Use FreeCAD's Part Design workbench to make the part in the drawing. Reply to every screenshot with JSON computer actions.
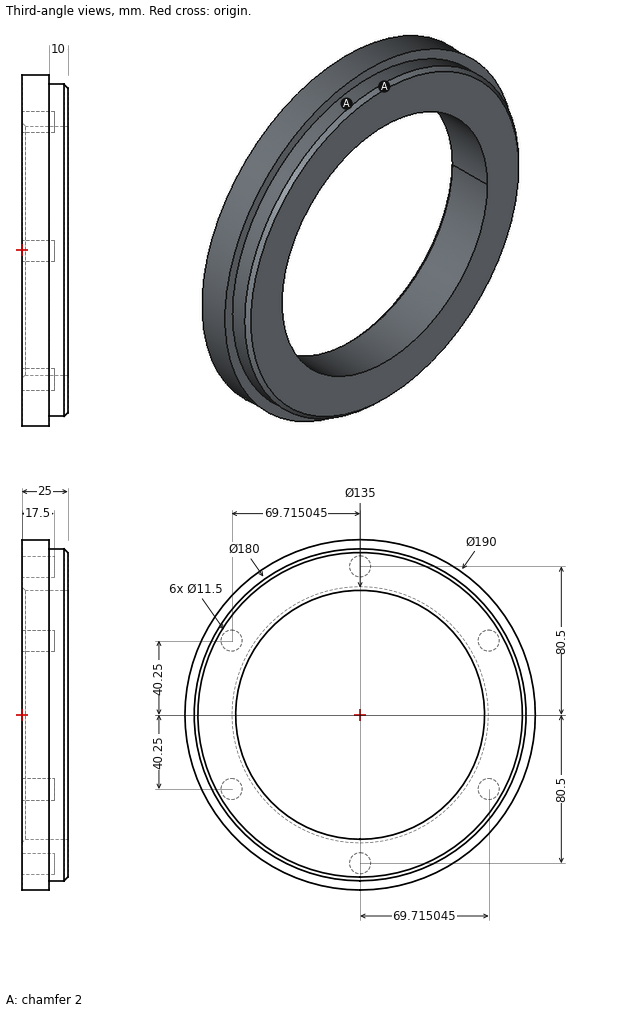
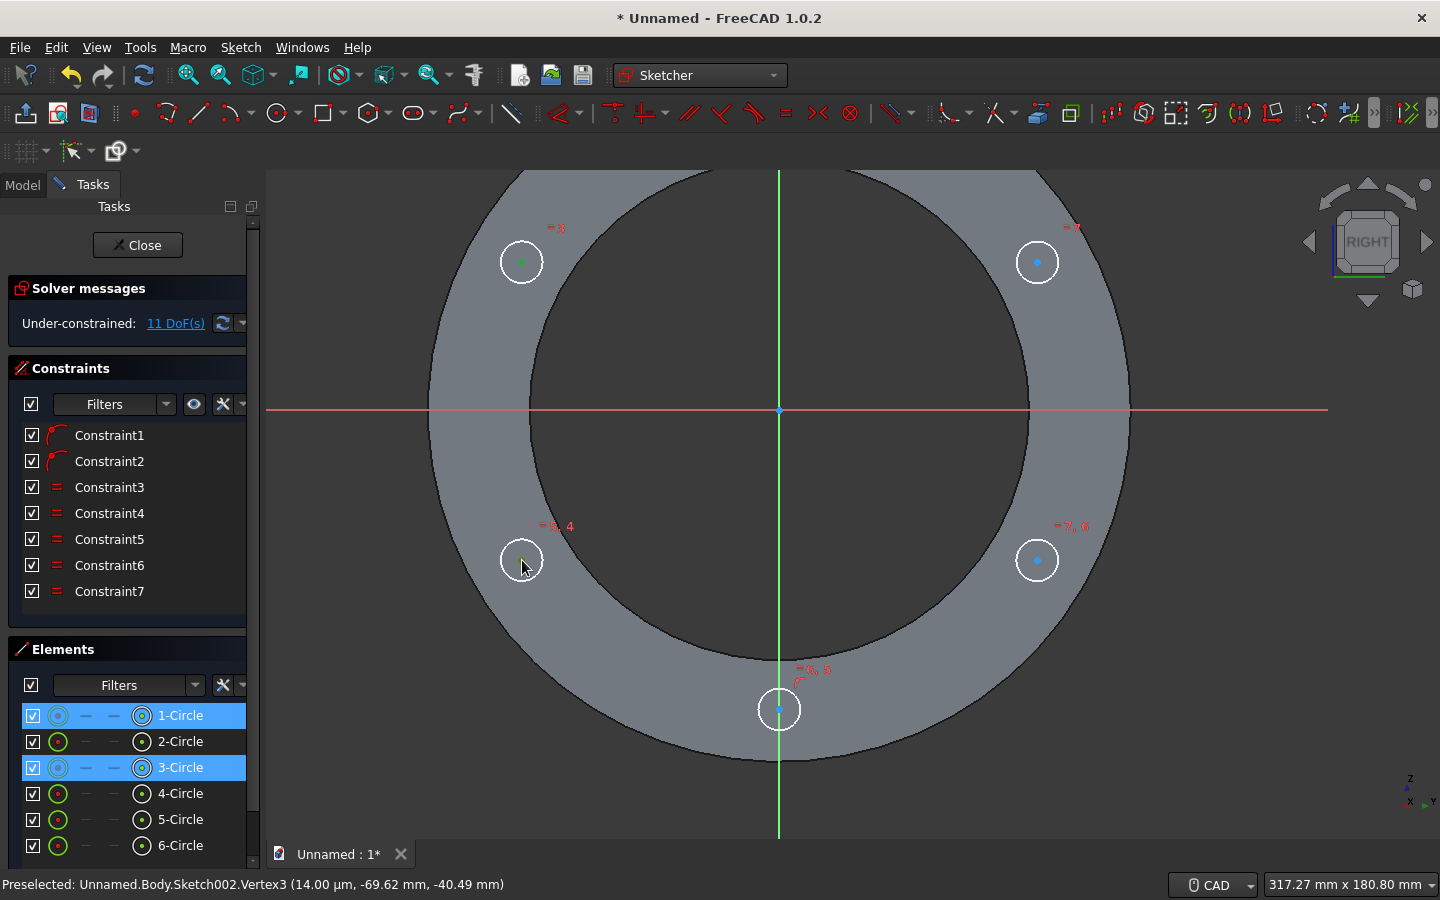
{"action": "key", "text": "v"}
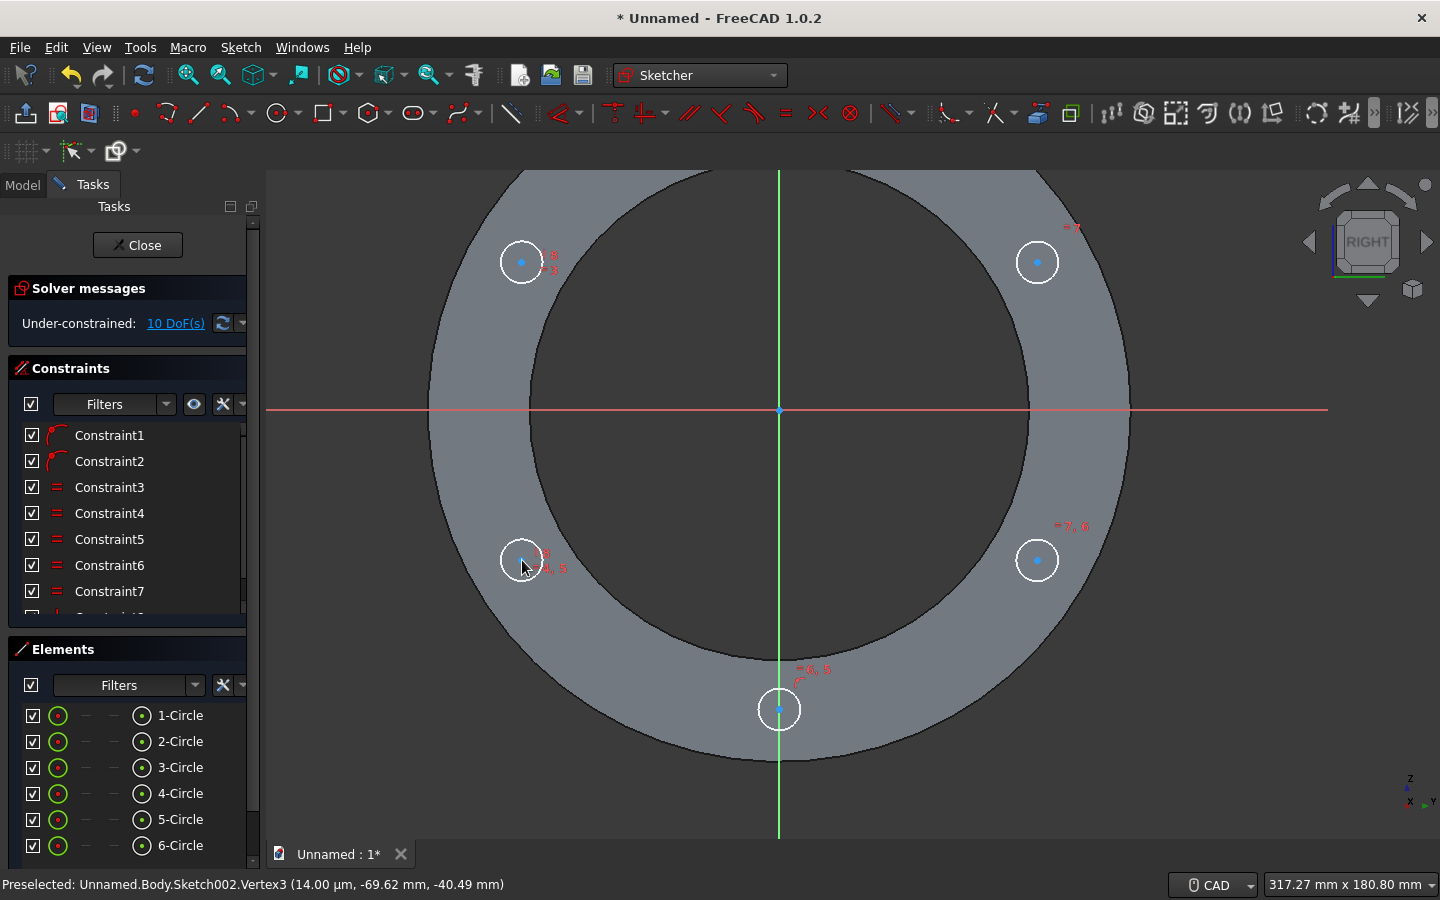
{"action": "left_click", "coordinate": [522, 560]}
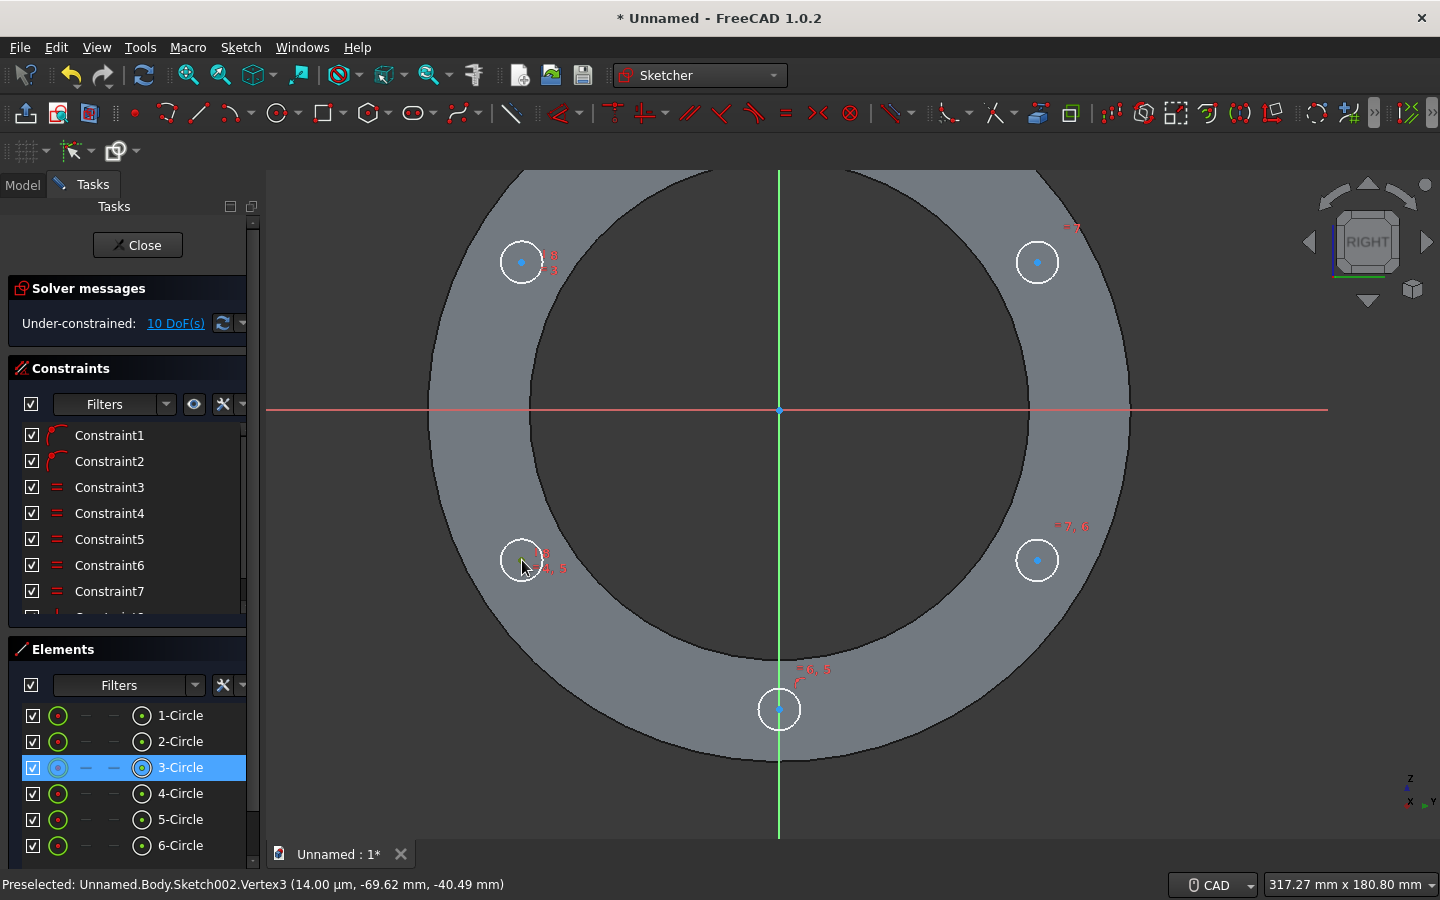
{"action": "left_click", "coordinate": [1037, 560]}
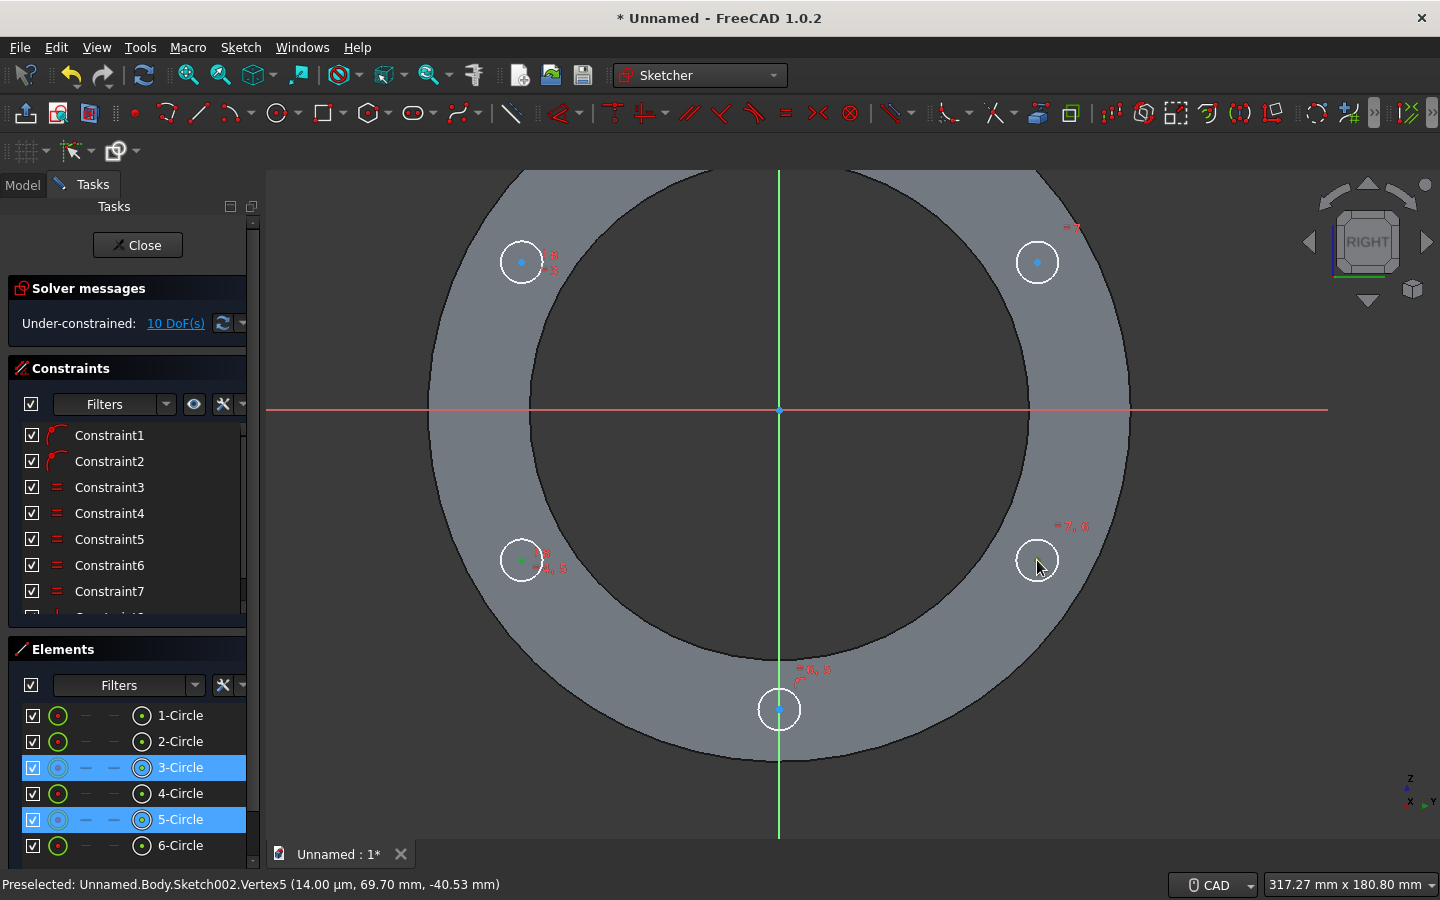
{"action": "left_click", "coordinate": [668, 114]}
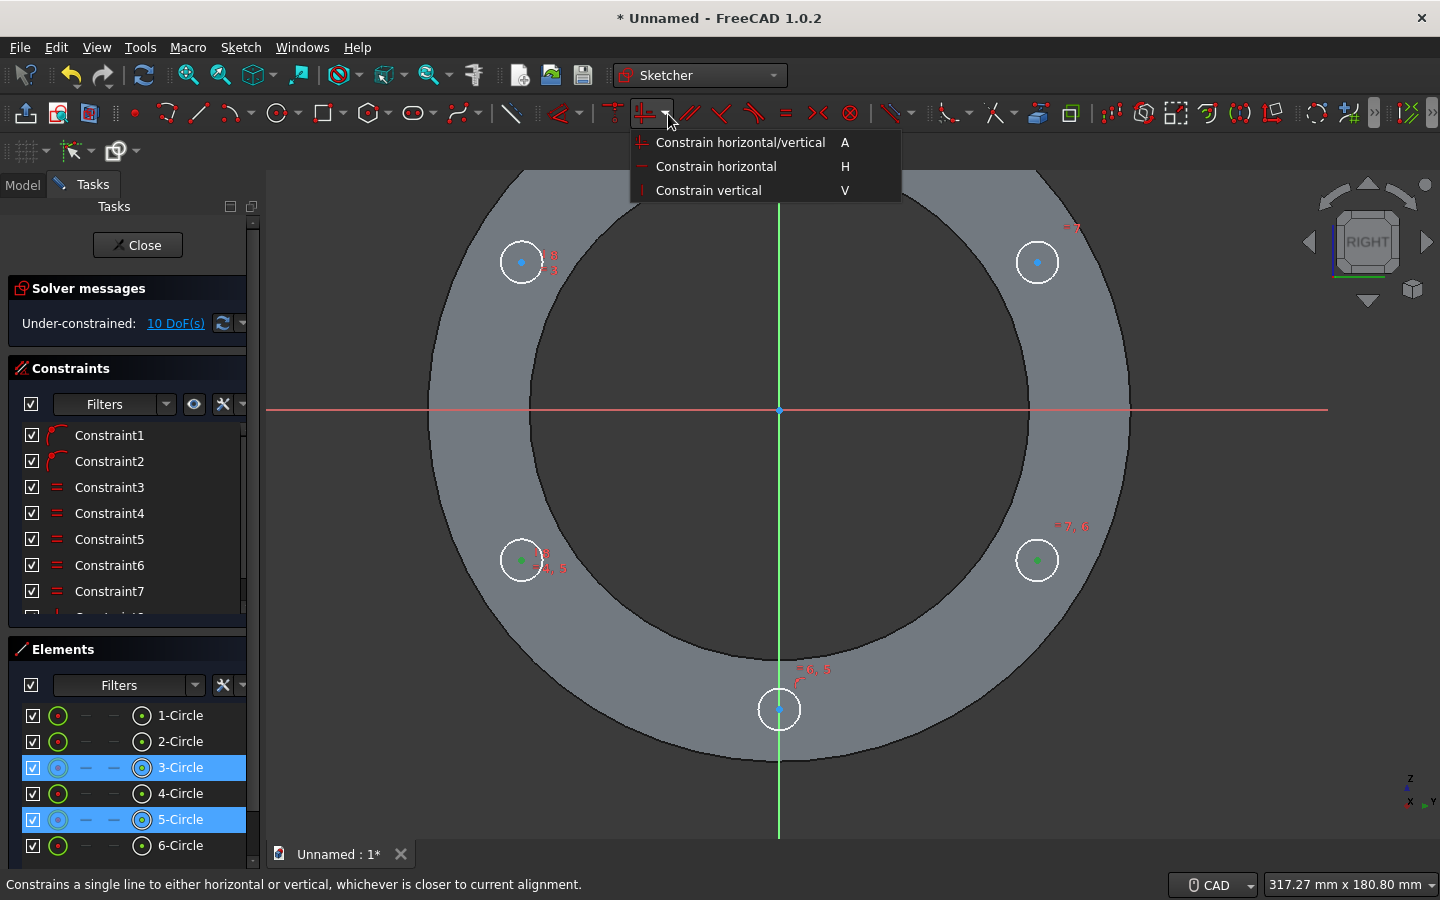
{"action": "left_click", "coordinate": [766, 166]}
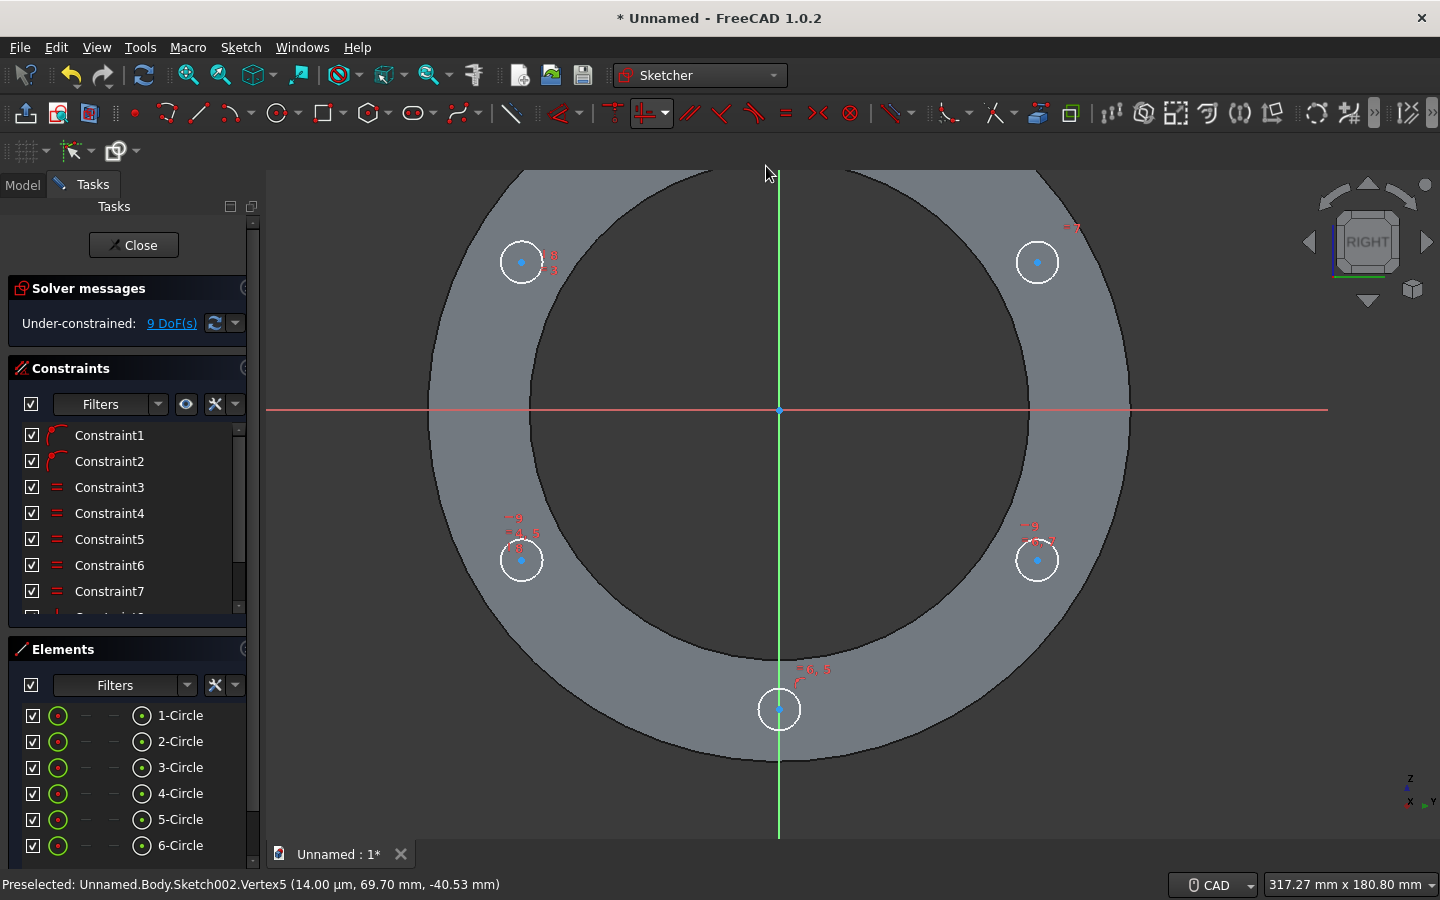
{"action": "left_click", "coordinate": [1037, 560]}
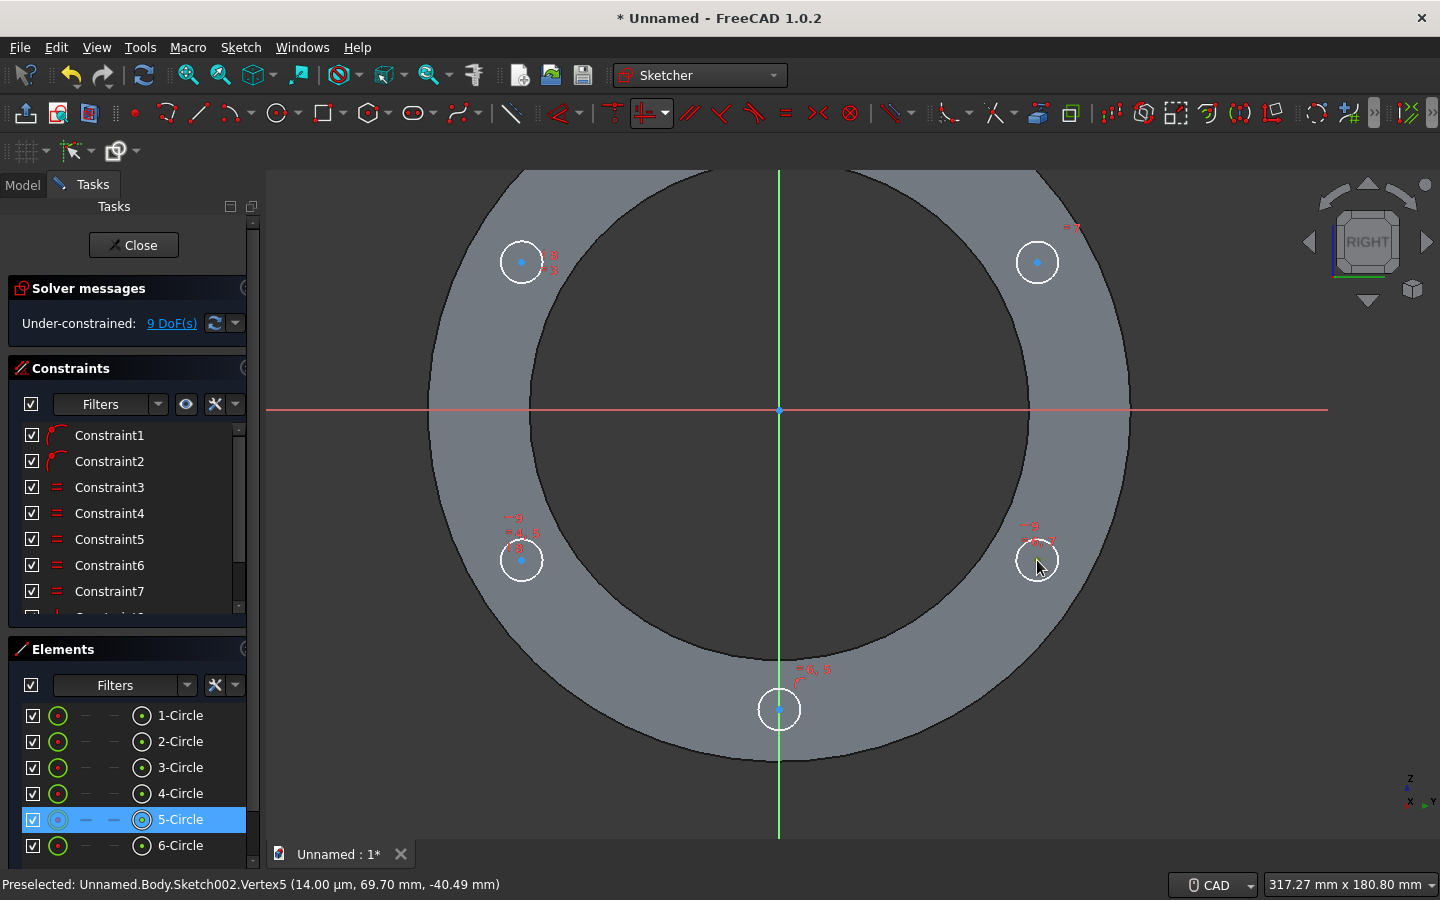
{"action": "left_click", "coordinate": [1038, 262]}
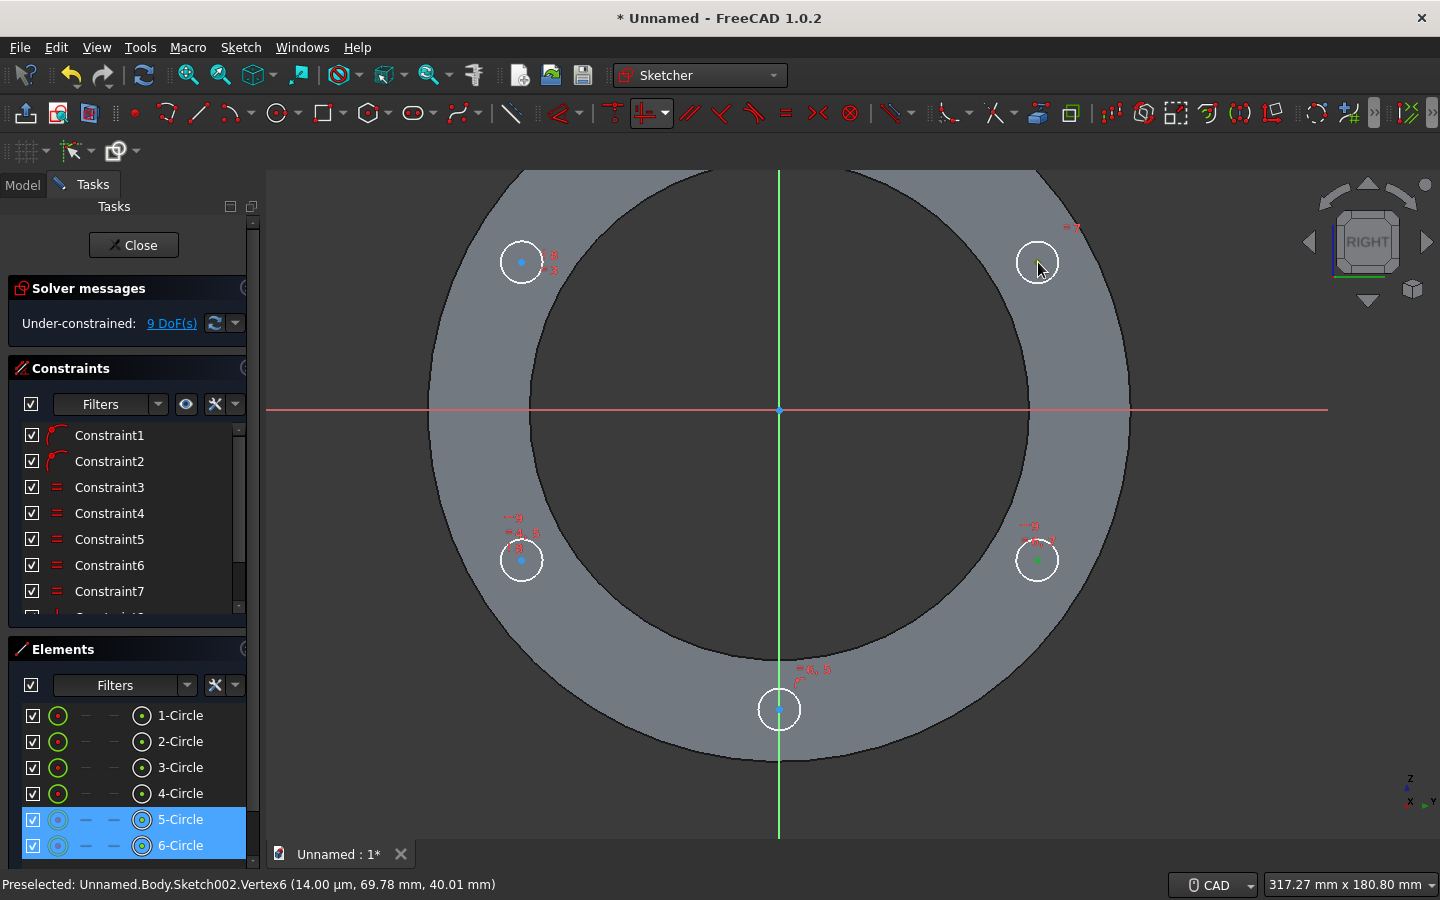
{"action": "key", "text": "v"}